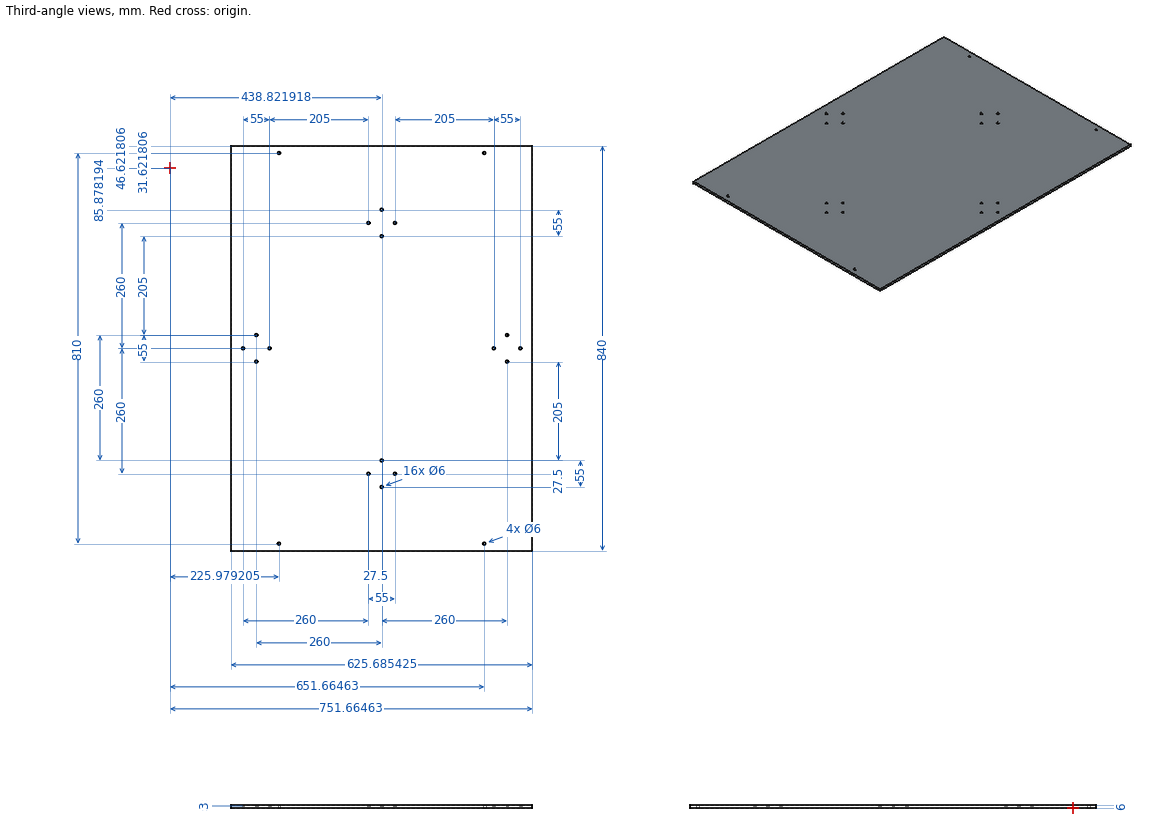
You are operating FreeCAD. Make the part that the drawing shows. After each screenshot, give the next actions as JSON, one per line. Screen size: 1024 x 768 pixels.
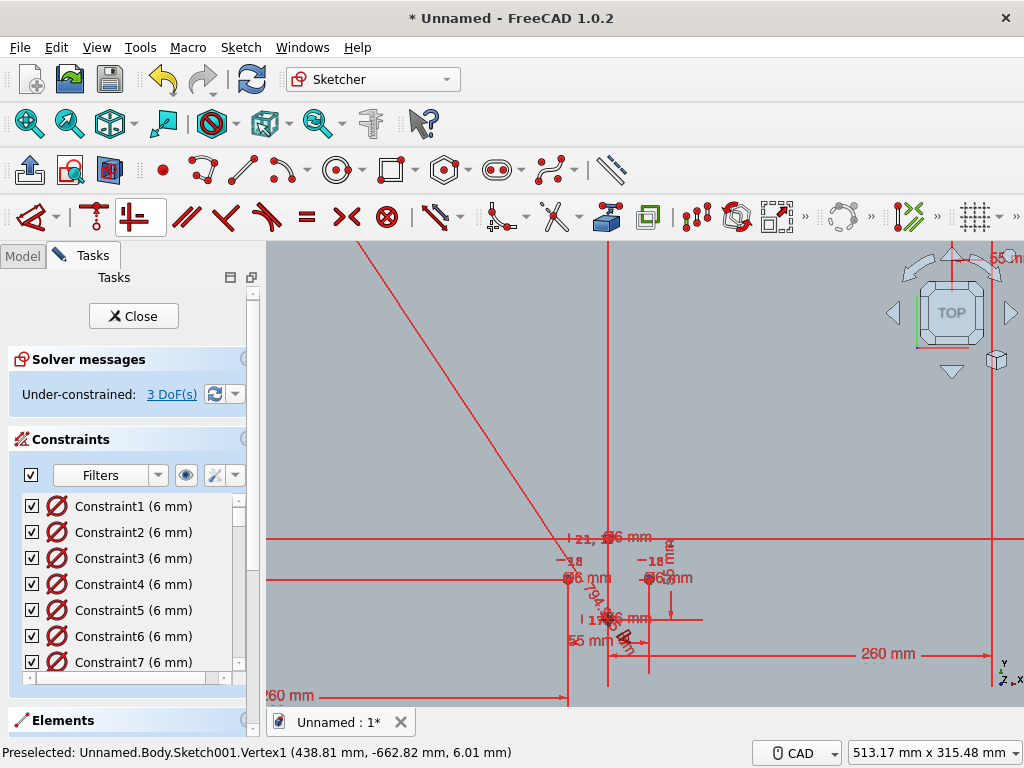
{"action": "left_click", "coordinate": [568, 580]}
{"action": "left_click", "coordinate": [588, 546]}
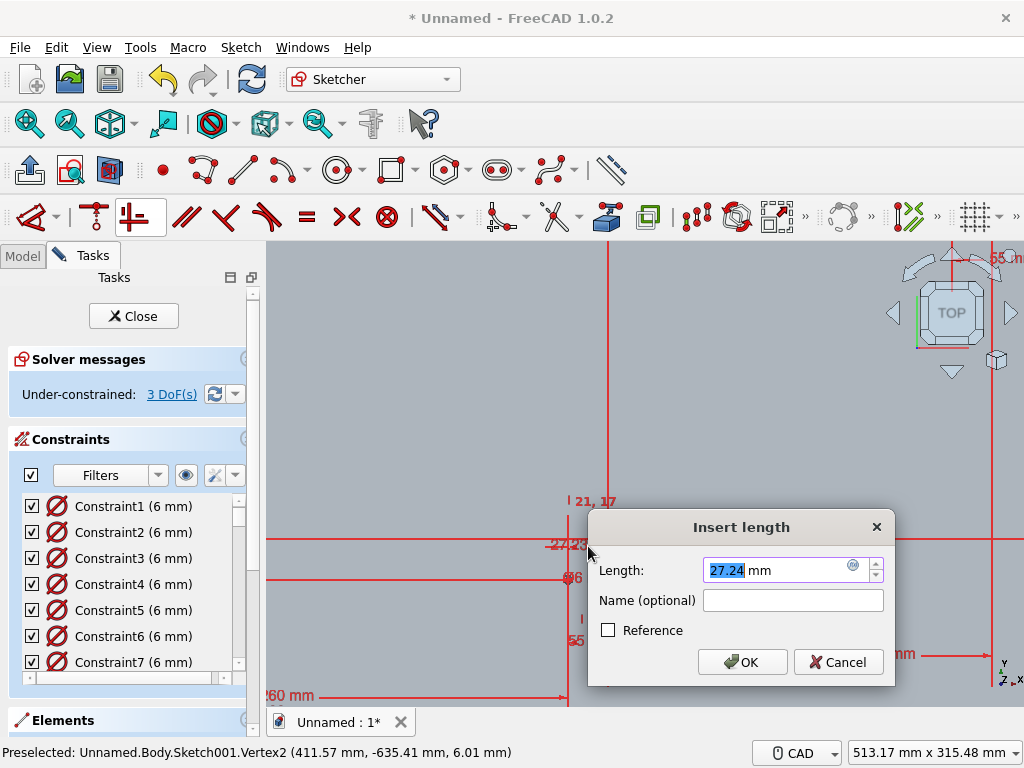
{"action": "type", "text": "27.5"}
{"action": "key", "text": "Return"}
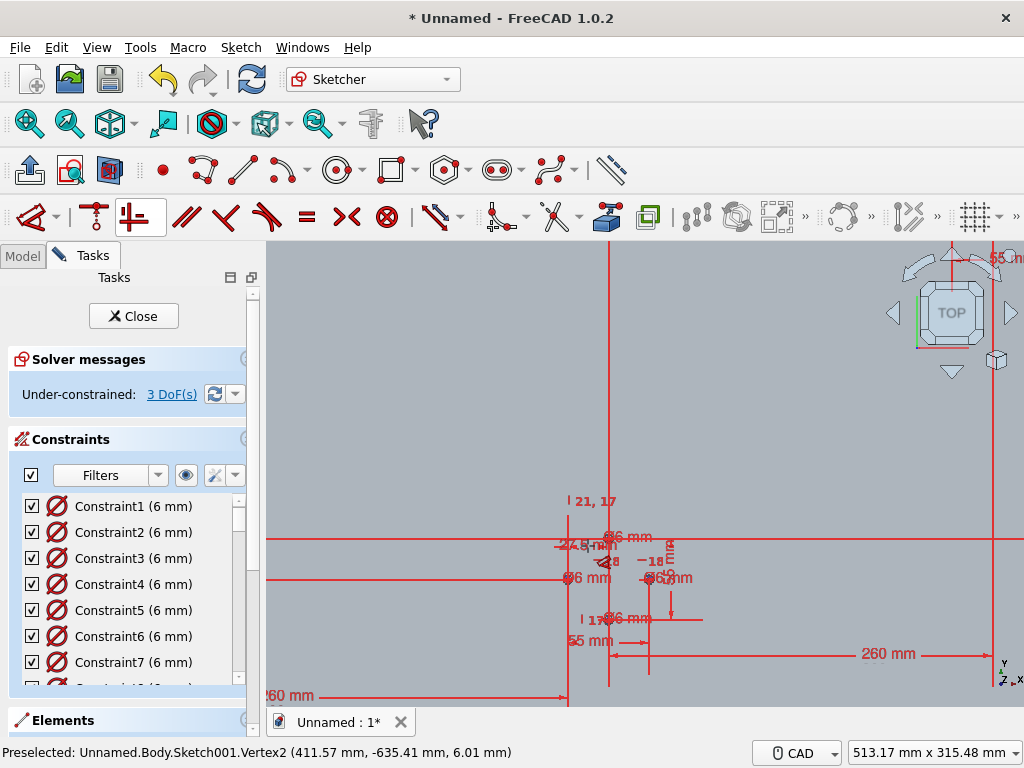
{"action": "left_click", "coordinate": [609, 620]}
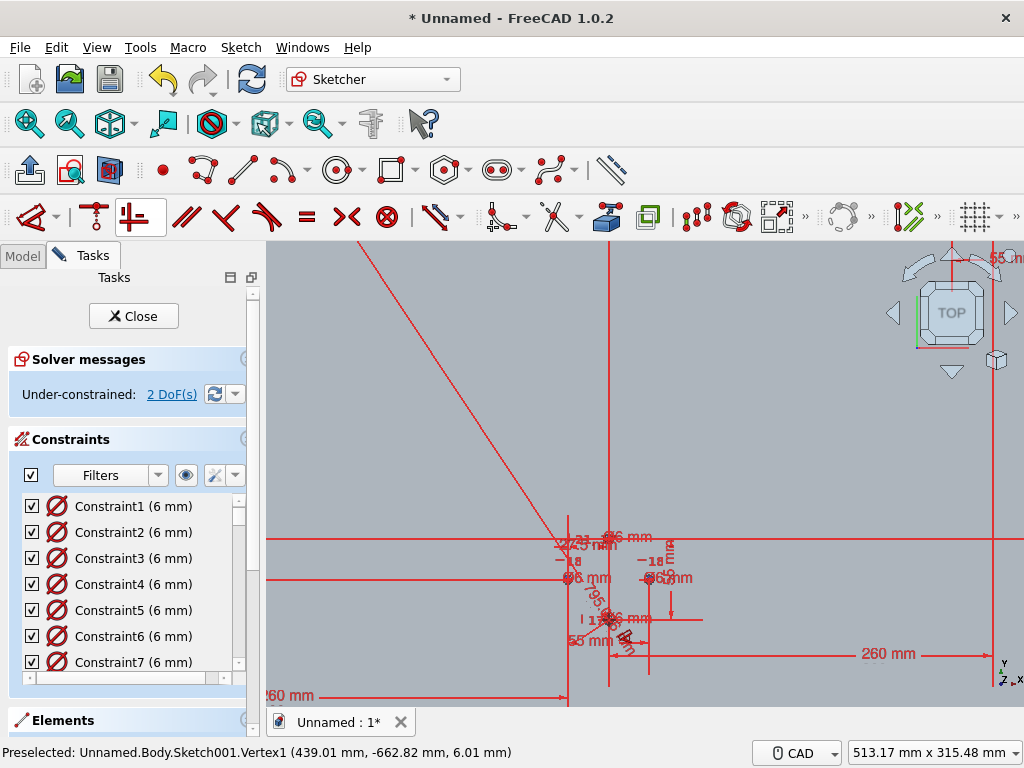
{"action": "left_click", "coordinate": [568, 580]}
{"action": "left_click", "coordinate": [643, 600]}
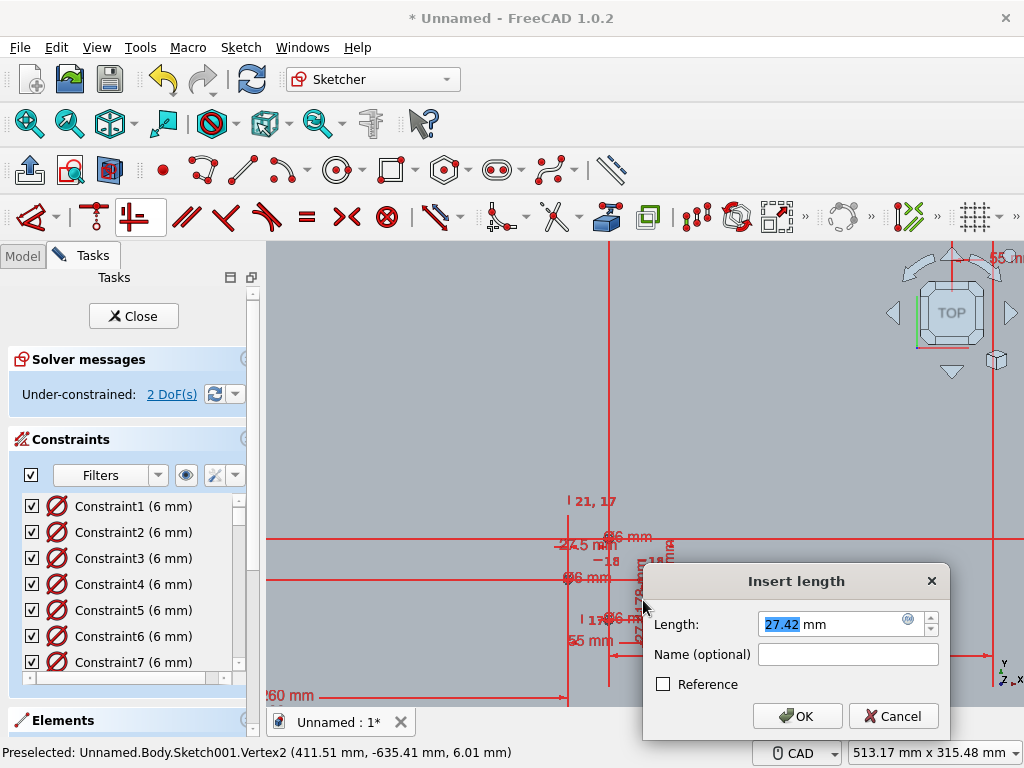
{"action": "type", "text": "27.5"}
{"action": "key", "text": "Return"}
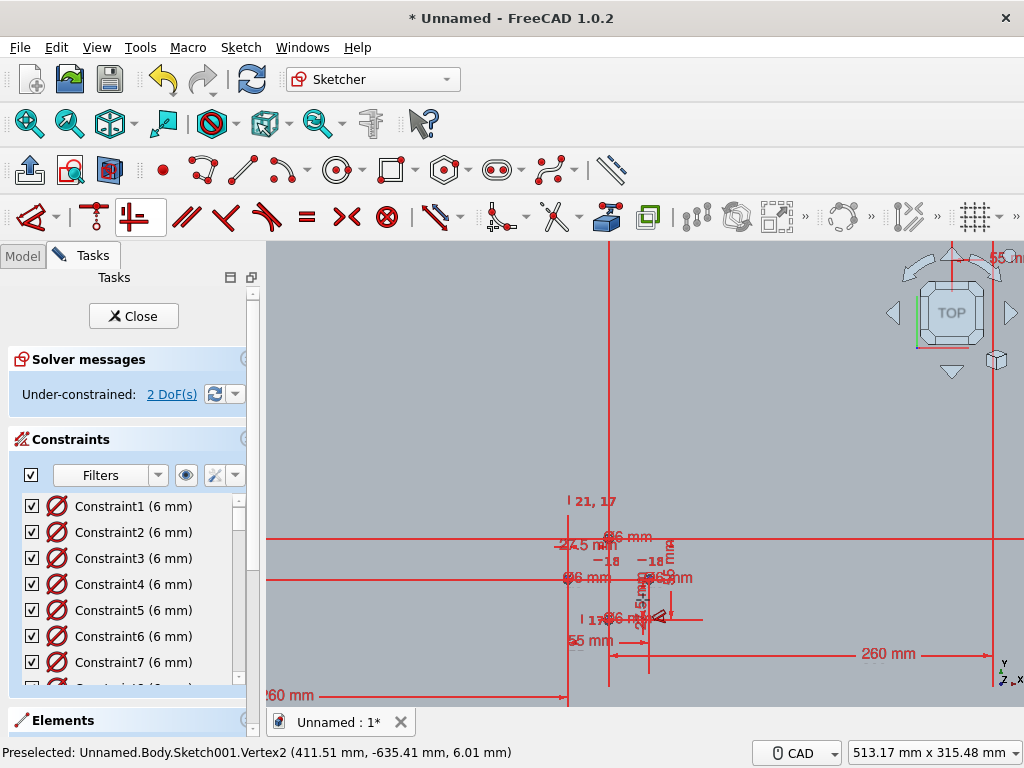
{"action": "scroll", "coordinate": [610, 622], "scroll_direction": "down", "scroll_amount": 6}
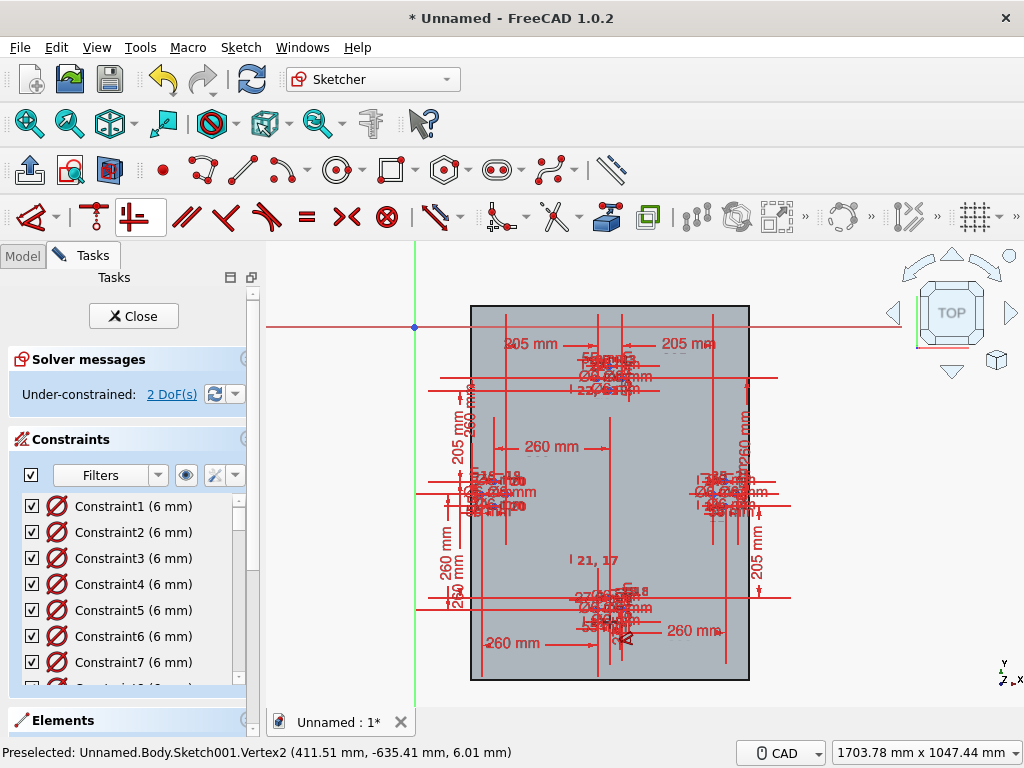
{"action": "left_click", "coordinate": [610, 366]}
{"action": "left_click", "coordinate": [381, 347]}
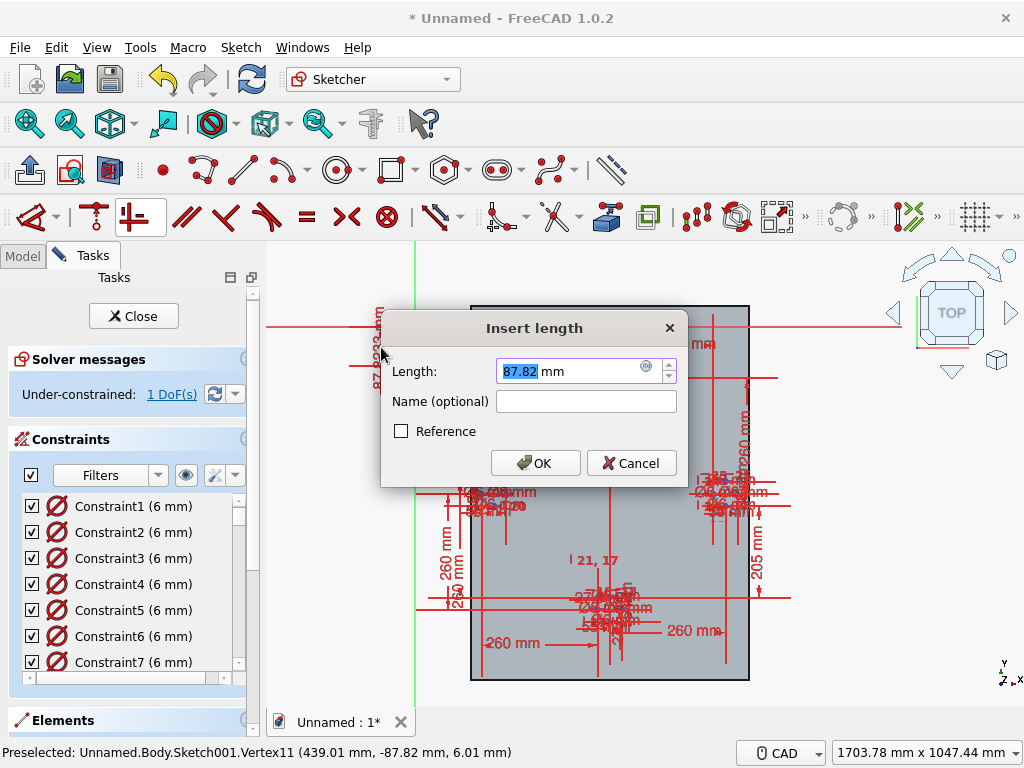
{"action": "type", "text": "85.878194"}
{"action": "key", "text": "Return"}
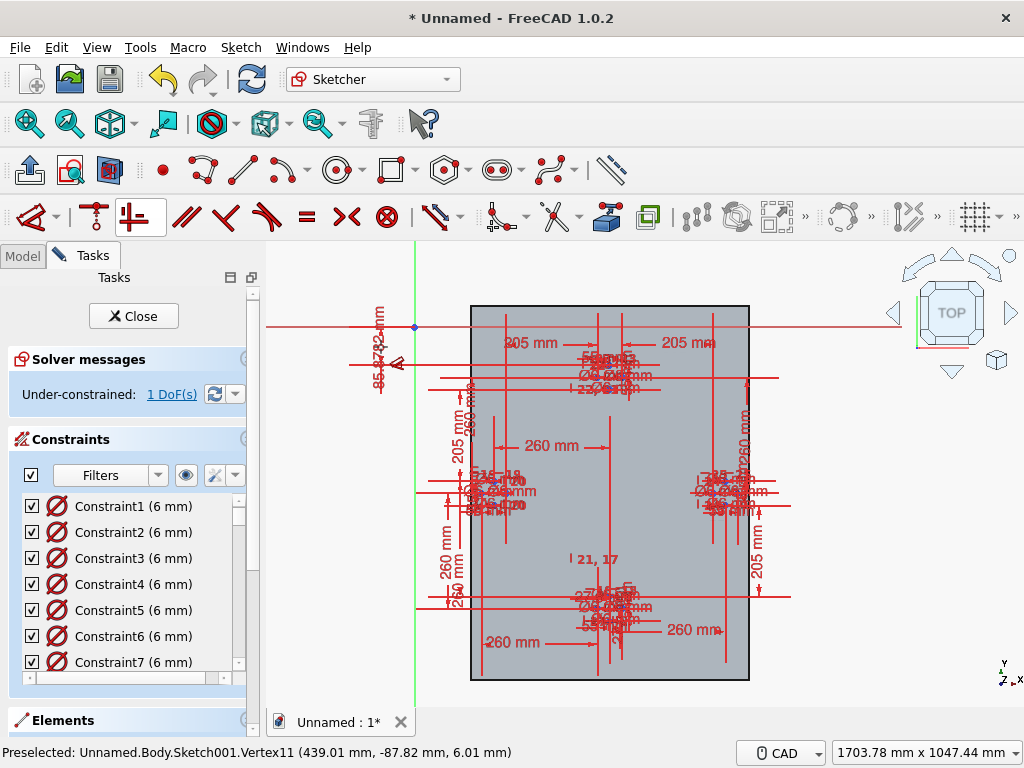
{"action": "left_click", "coordinate": [610, 621]}
{"action": "left_click", "coordinate": [512, 293]}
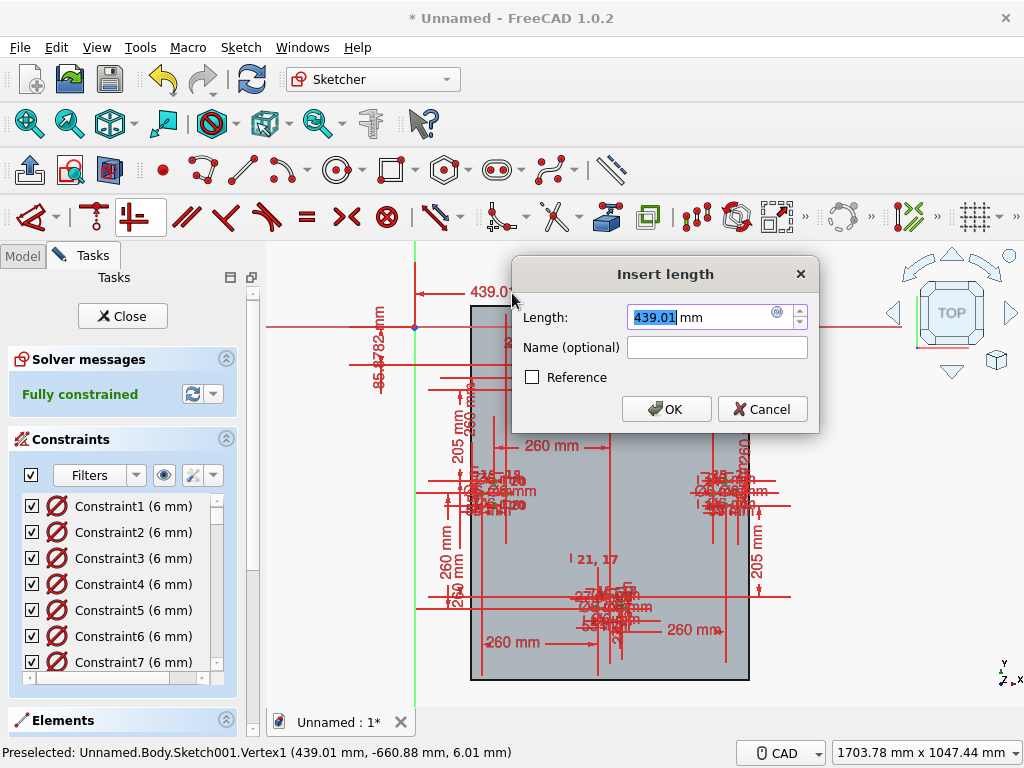
{"action": "type", "text": "438.821918"}
{"action": "key", "text": "Return"}
{"action": "key", "text": "Escape"}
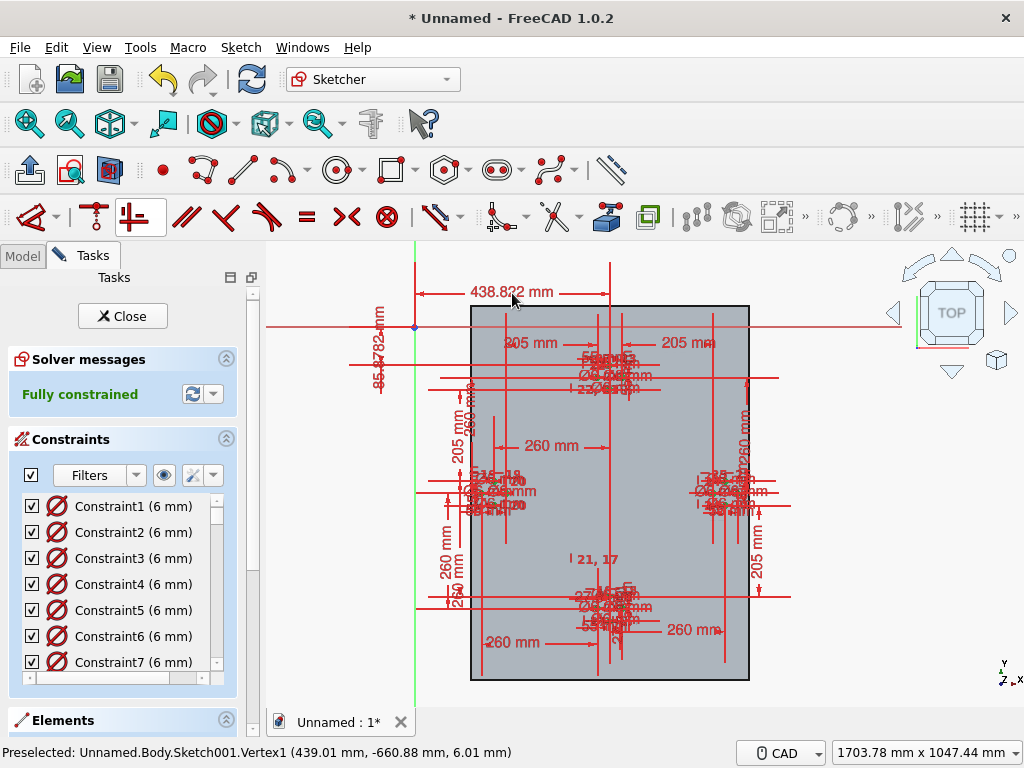
{"action": "left_click", "coordinate": [123, 316]}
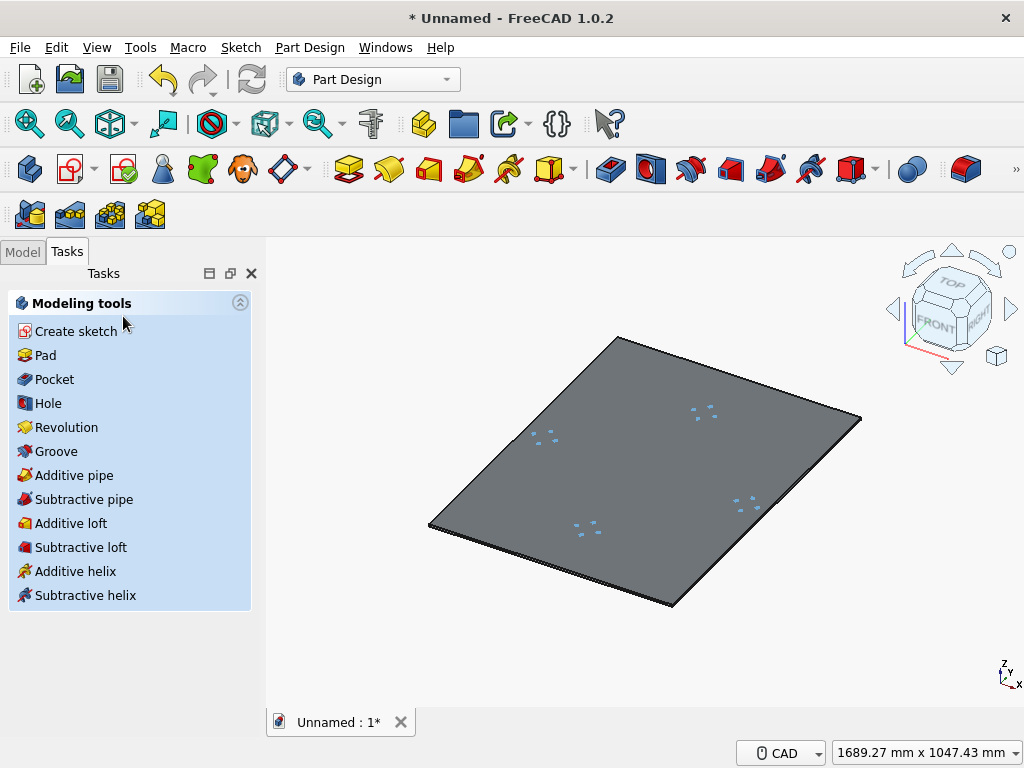
{"action": "left_click", "coordinate": [612, 170]}